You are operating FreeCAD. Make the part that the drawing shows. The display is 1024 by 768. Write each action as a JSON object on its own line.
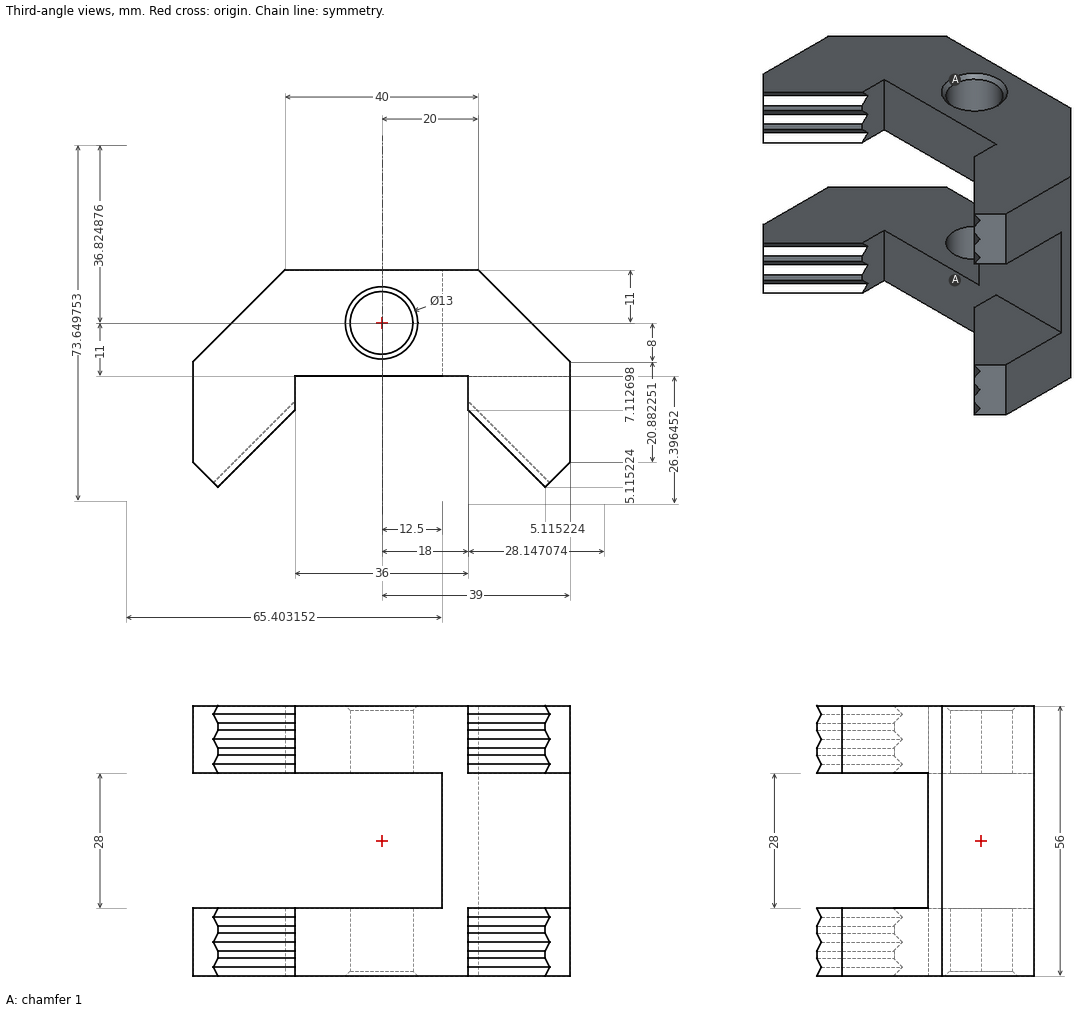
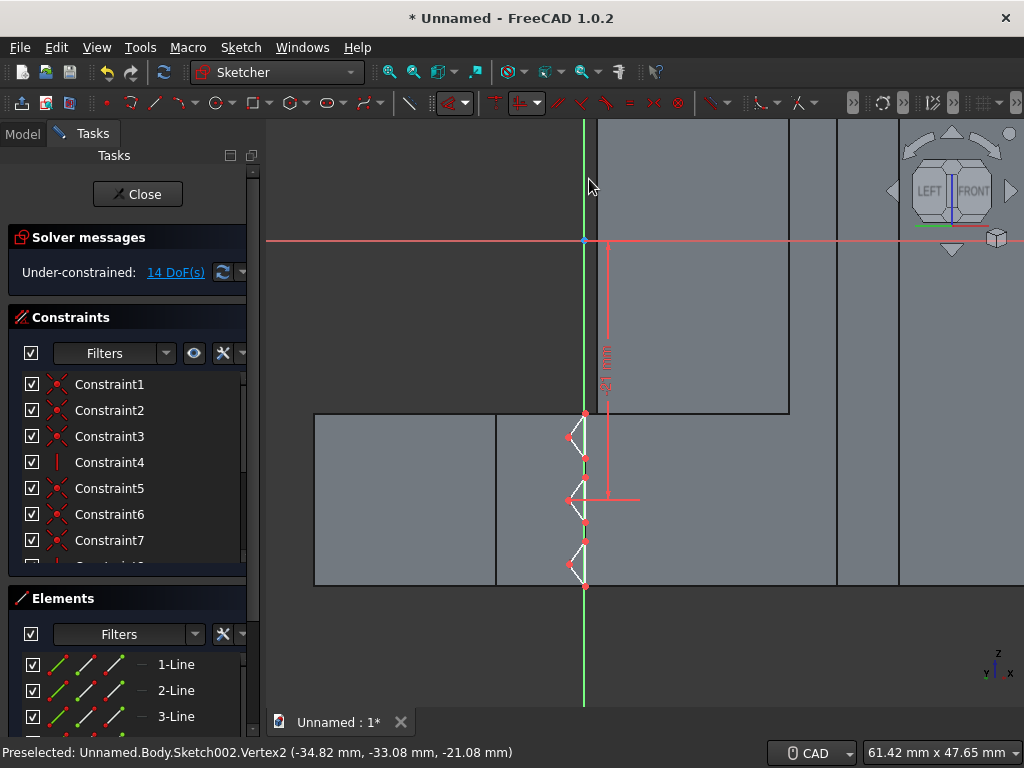
{"action": "left_click", "coordinate": [585, 414]}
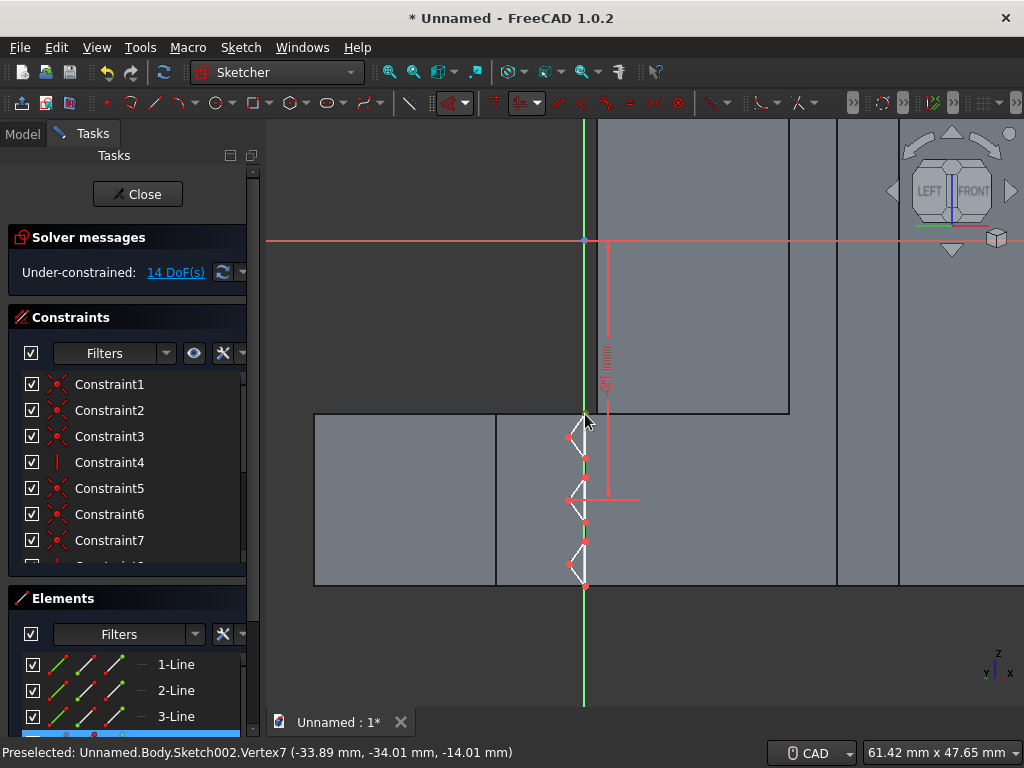
{"action": "left_click", "coordinate": [468, 104]}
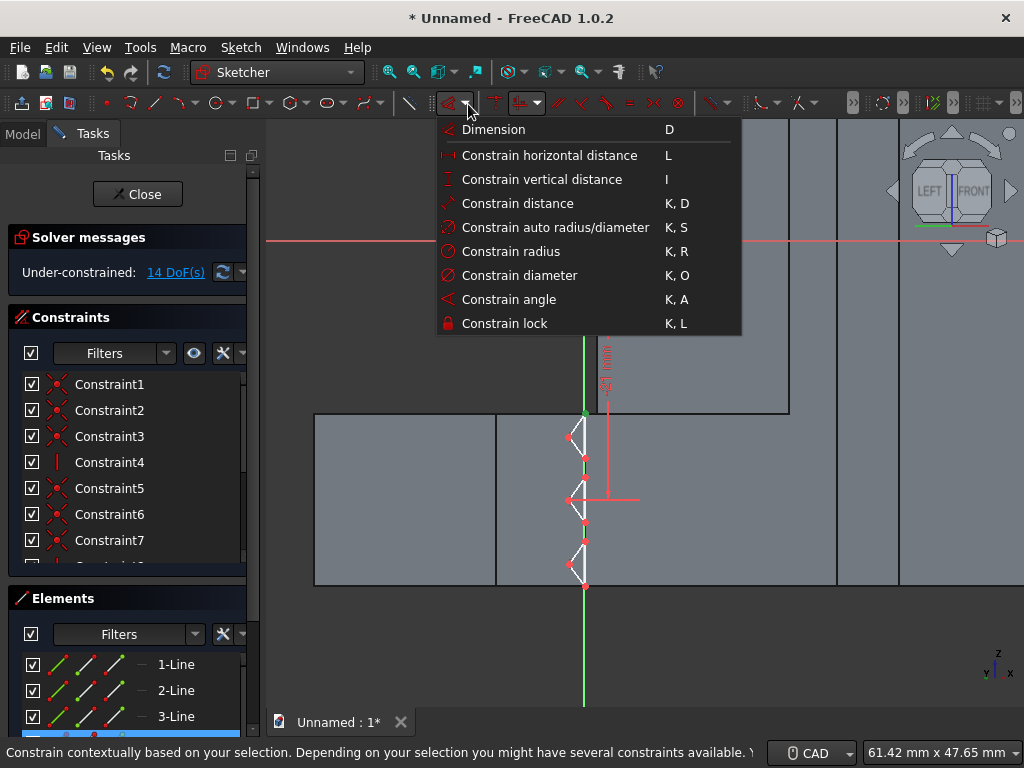
{"action": "left_click", "coordinate": [589, 179]}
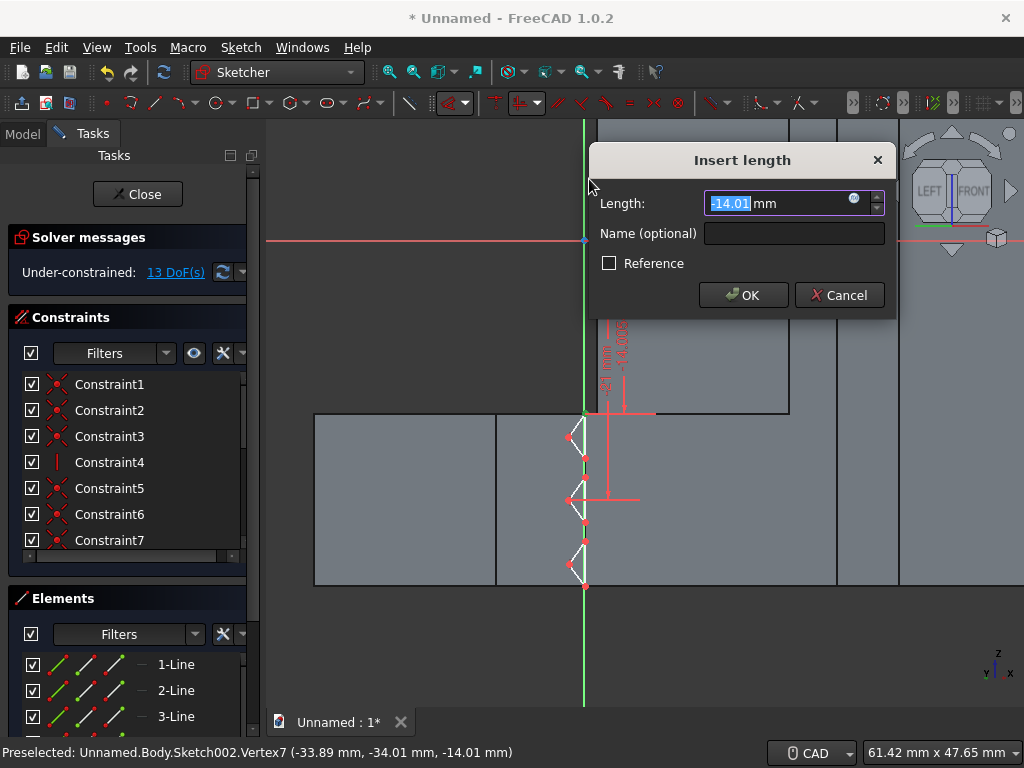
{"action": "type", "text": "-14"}
{"action": "key", "text": "Return"}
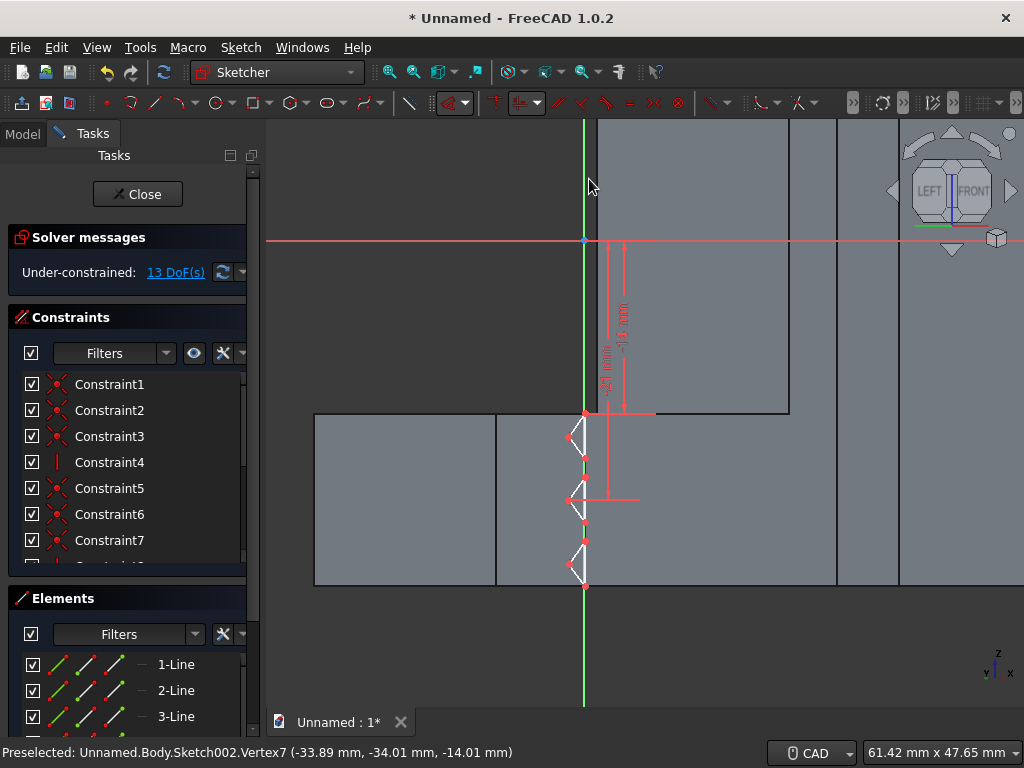
{"action": "left_click", "coordinate": [585, 587]}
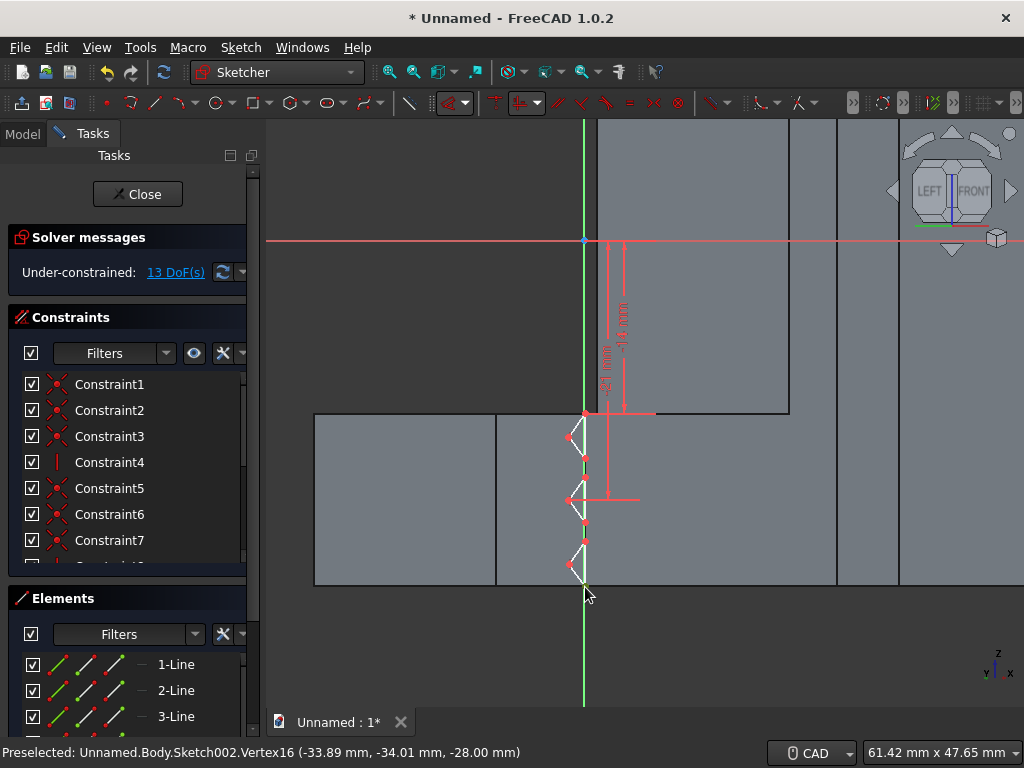
{"action": "left_click", "coordinate": [468, 104]}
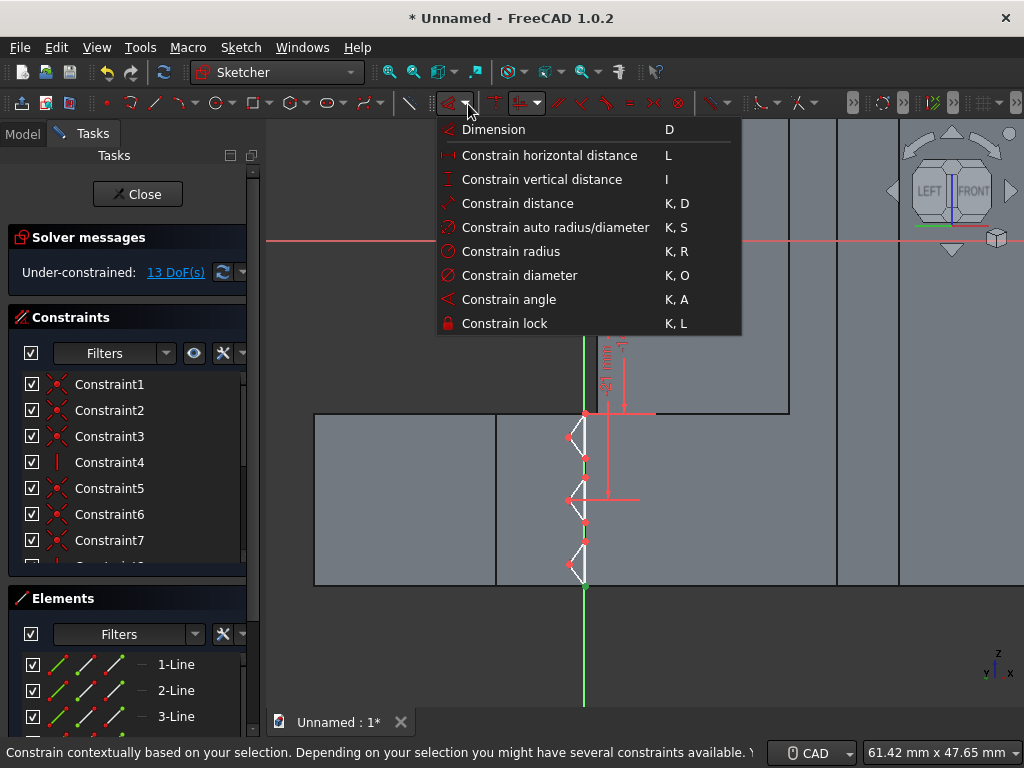
{"action": "left_click", "coordinate": [589, 179]}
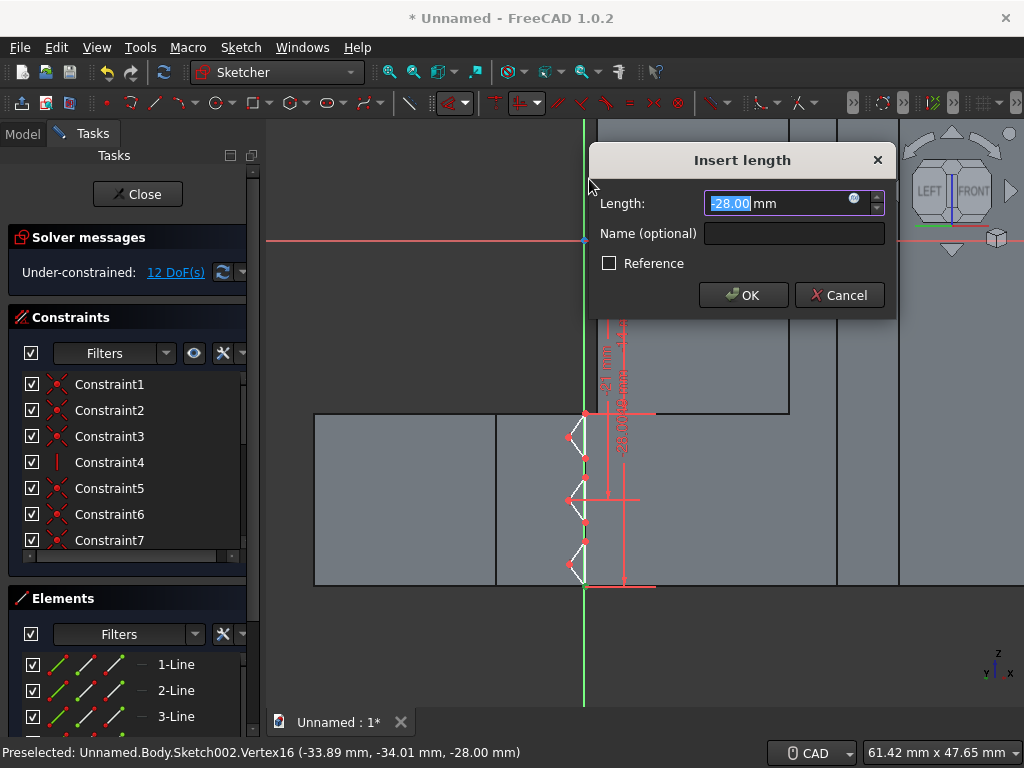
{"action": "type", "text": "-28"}
{"action": "key", "text": "Return"}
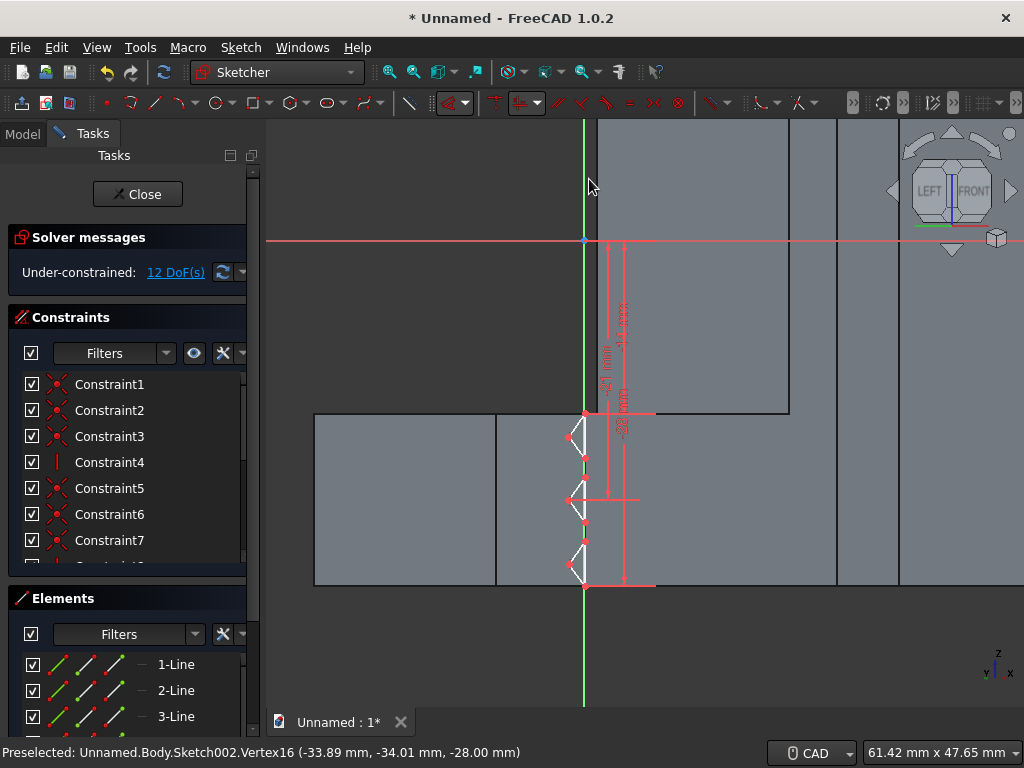
{"action": "scroll", "coordinate": [585, 505], "scroll_direction": "up", "scroll_amount": 2}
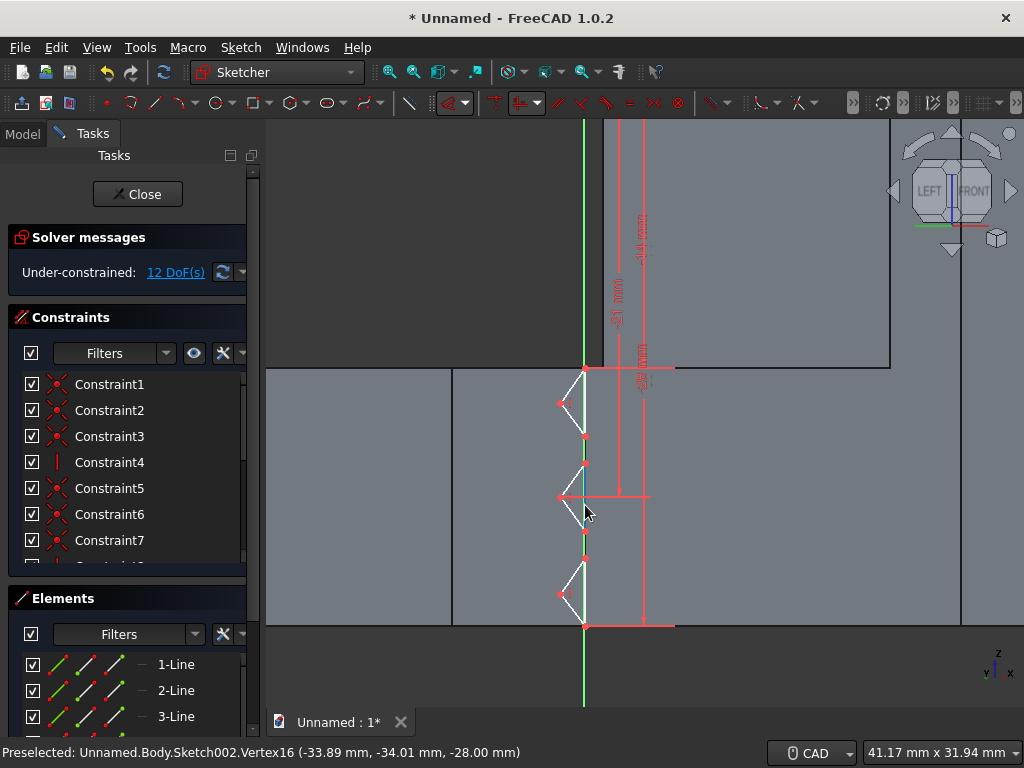
{"action": "left_click", "coordinate": [585, 504]}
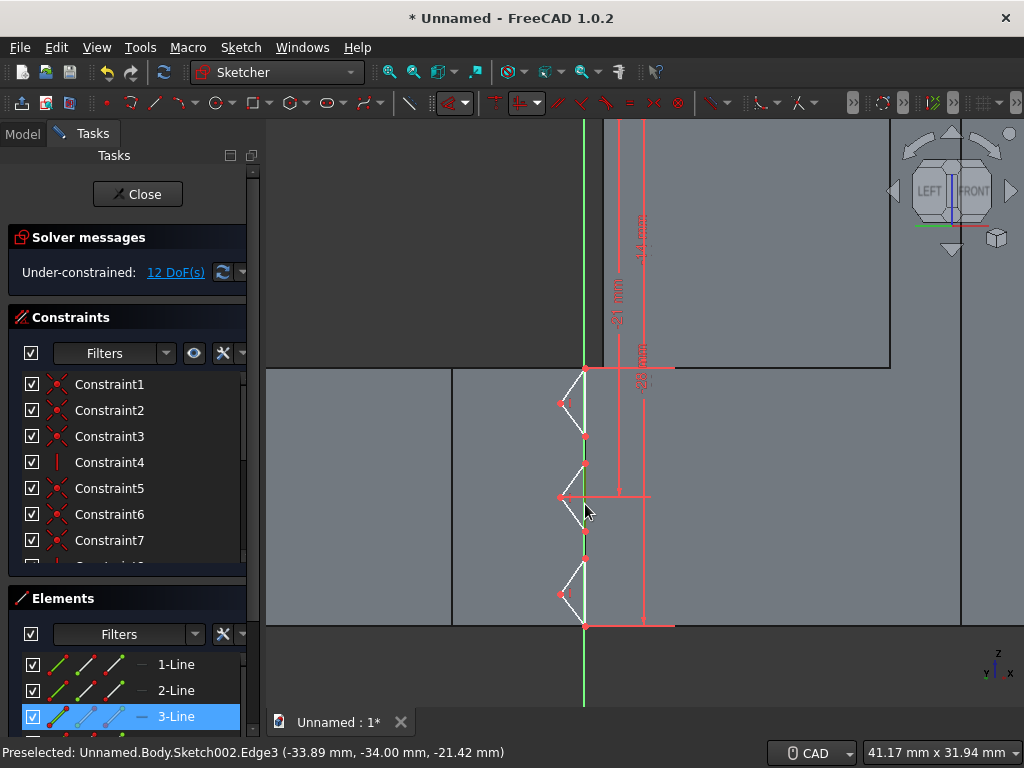
{"action": "left_click", "coordinate": [468, 104]}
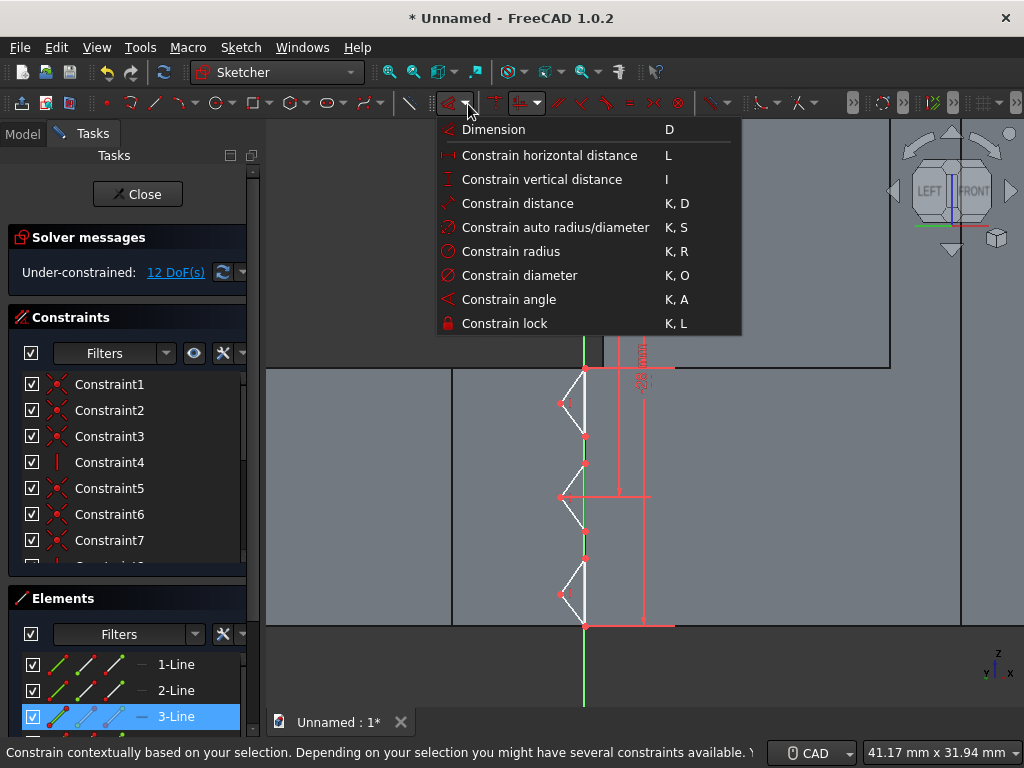
{"action": "left_click", "coordinate": [589, 179]}